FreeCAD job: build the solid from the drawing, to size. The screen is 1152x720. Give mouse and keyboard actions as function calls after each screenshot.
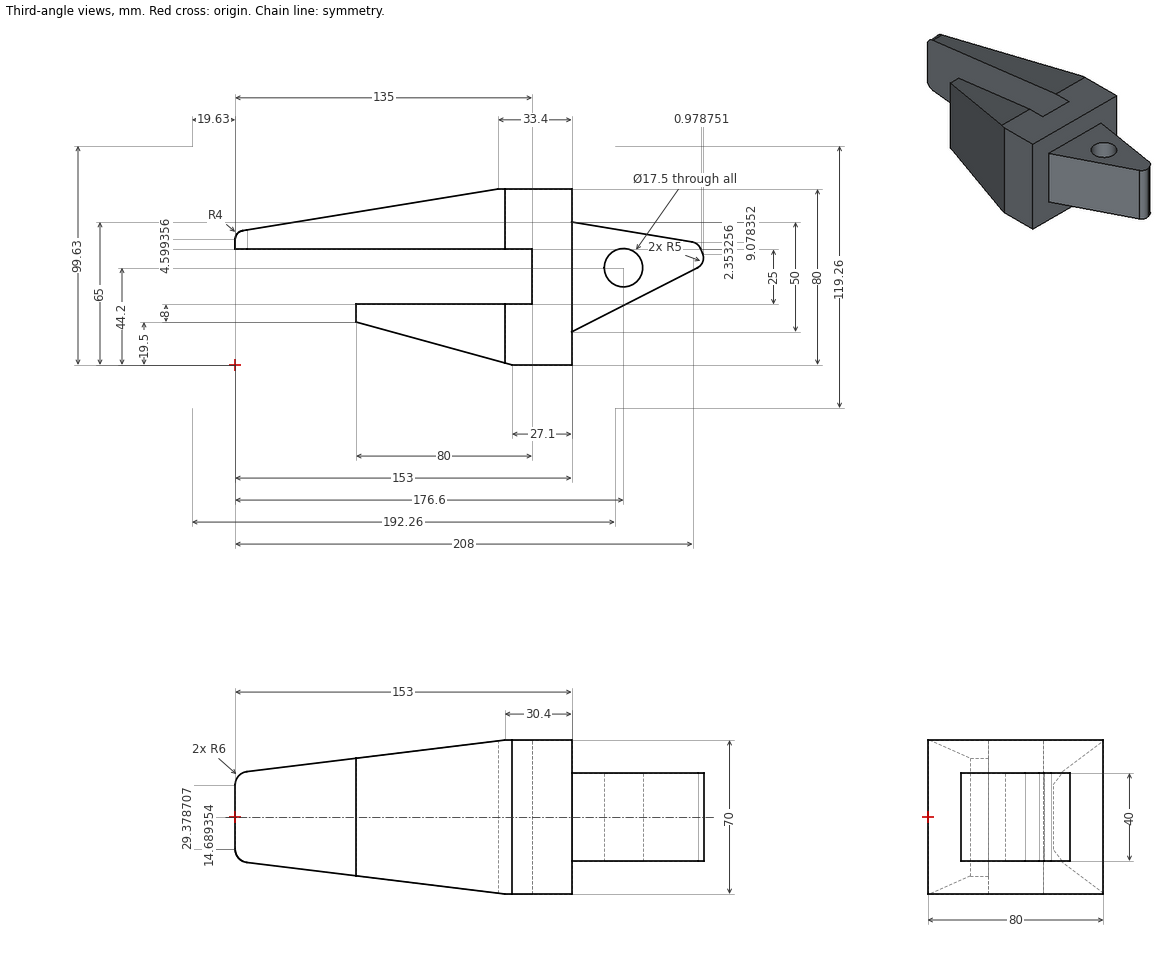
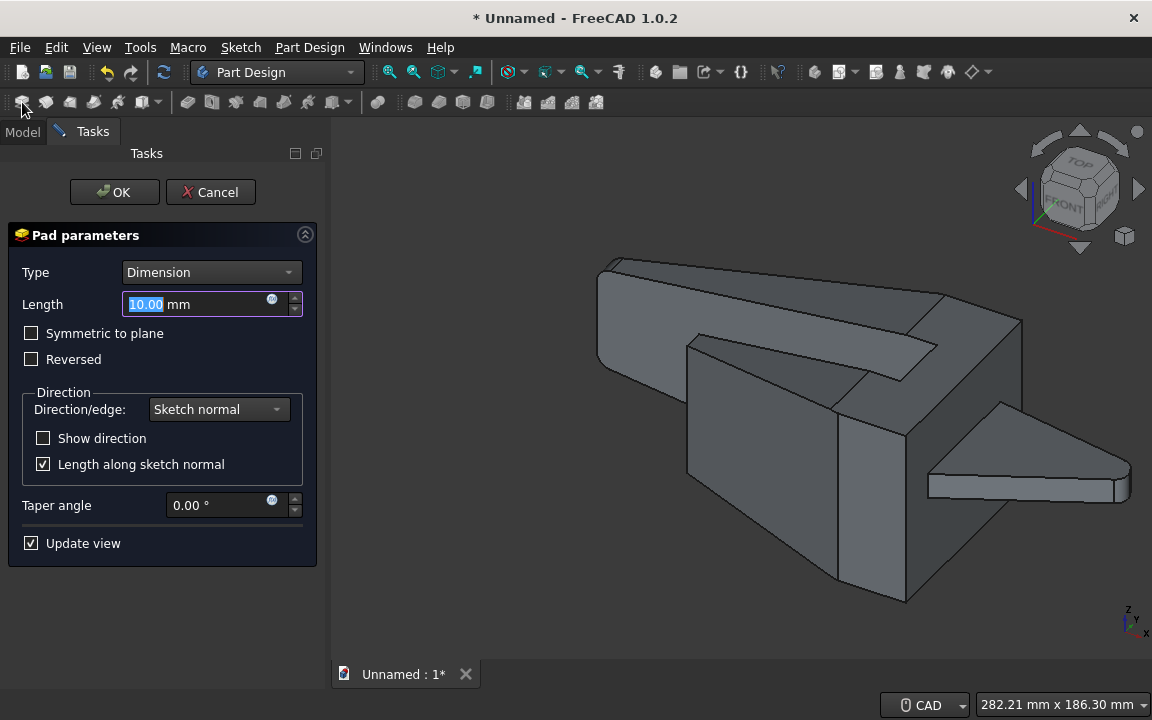
text(40)
key(Tab)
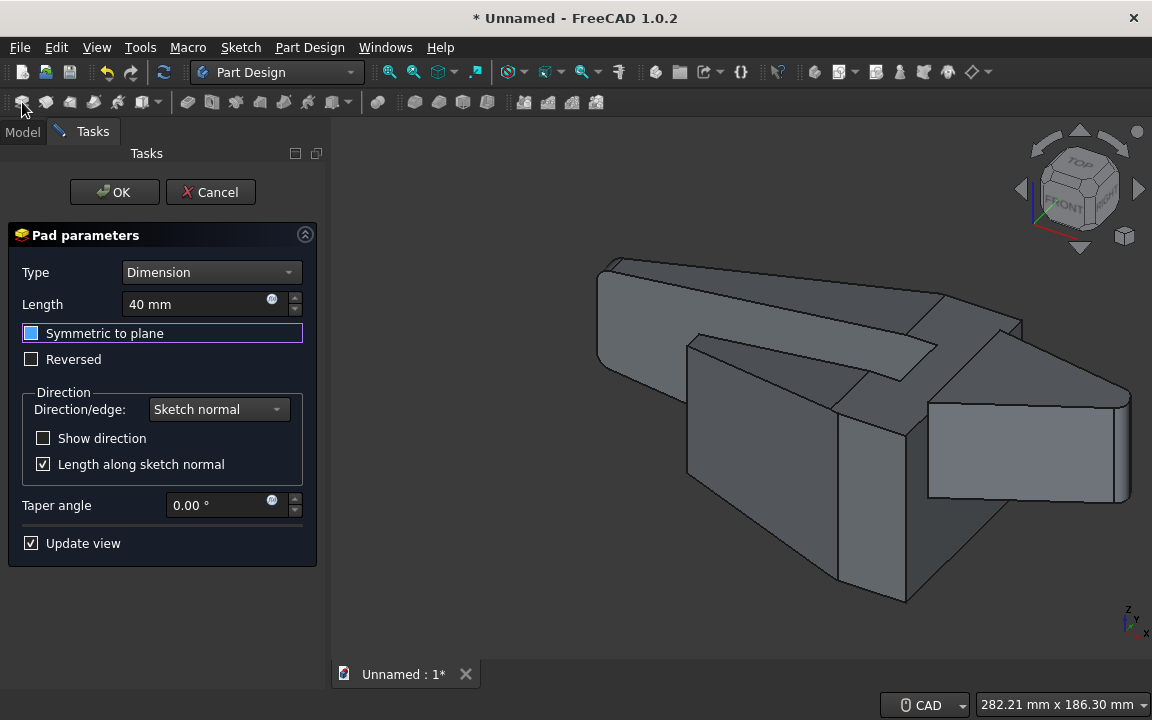
click(30, 333)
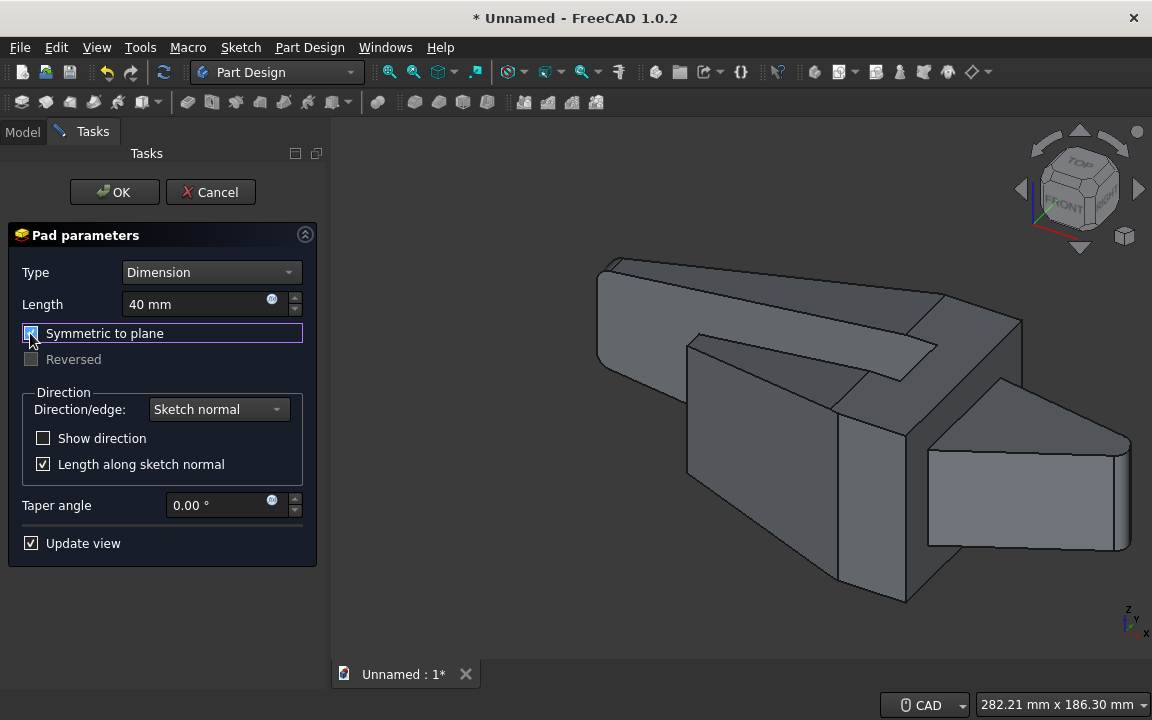
click(115, 192)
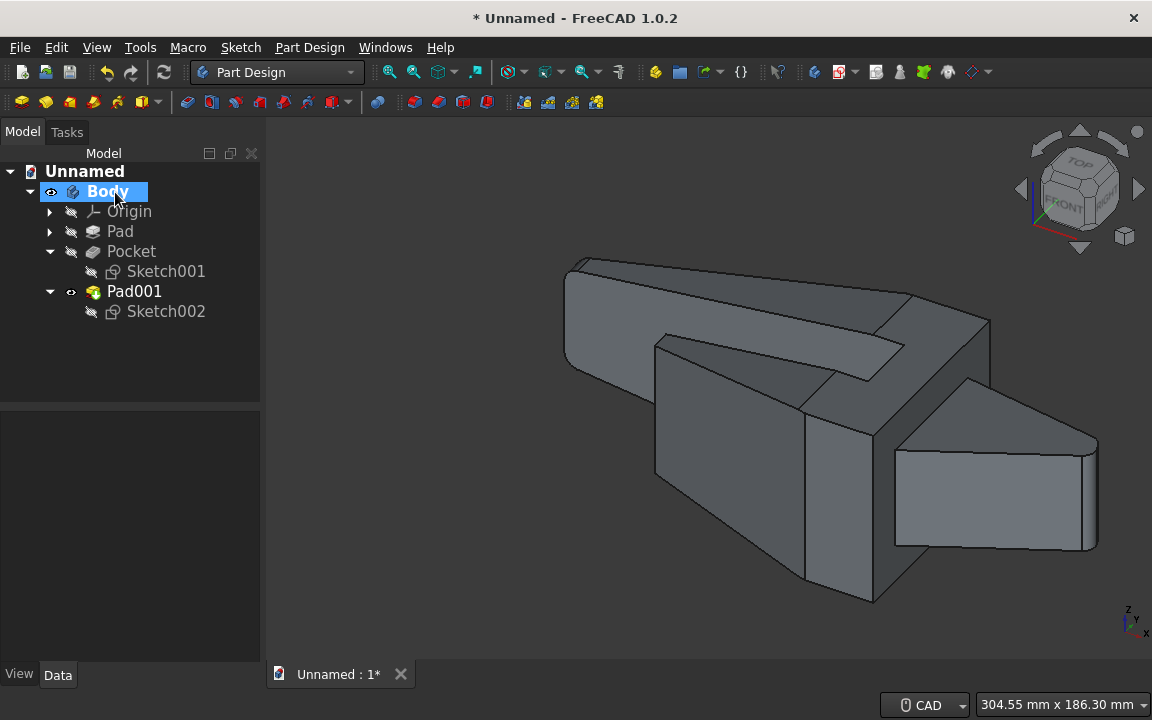
click(996, 421)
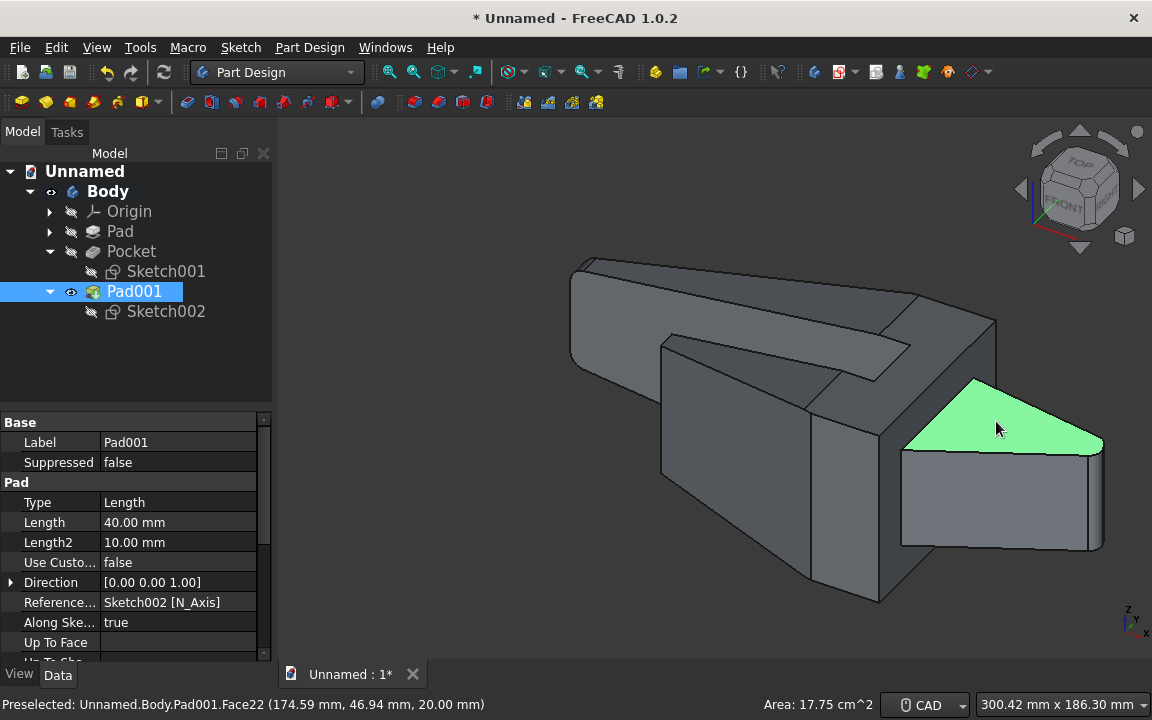
click(840, 72)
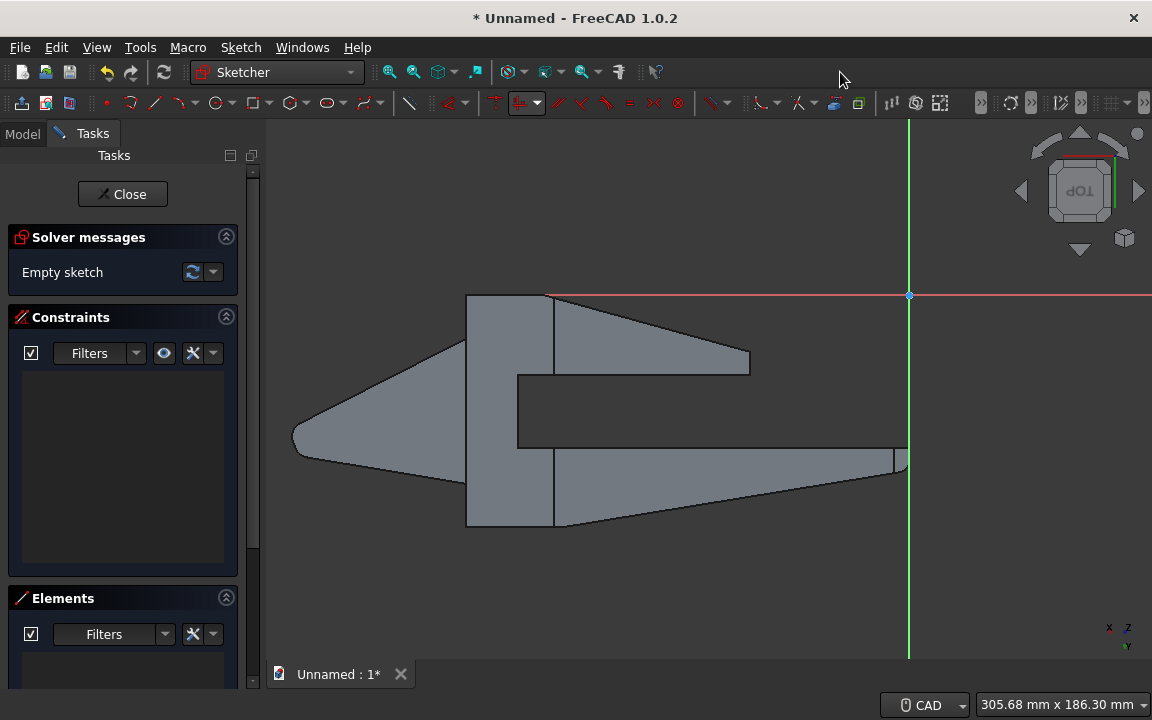
key(q)
key(s)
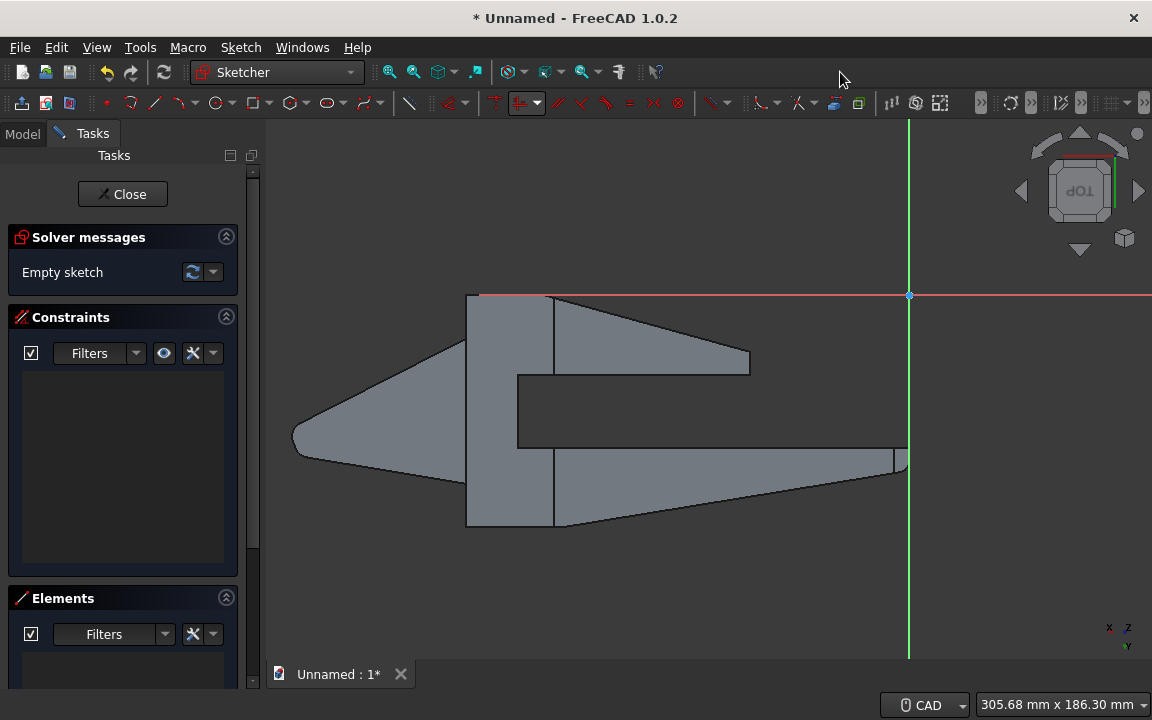
scroll(359, 429, up, 10)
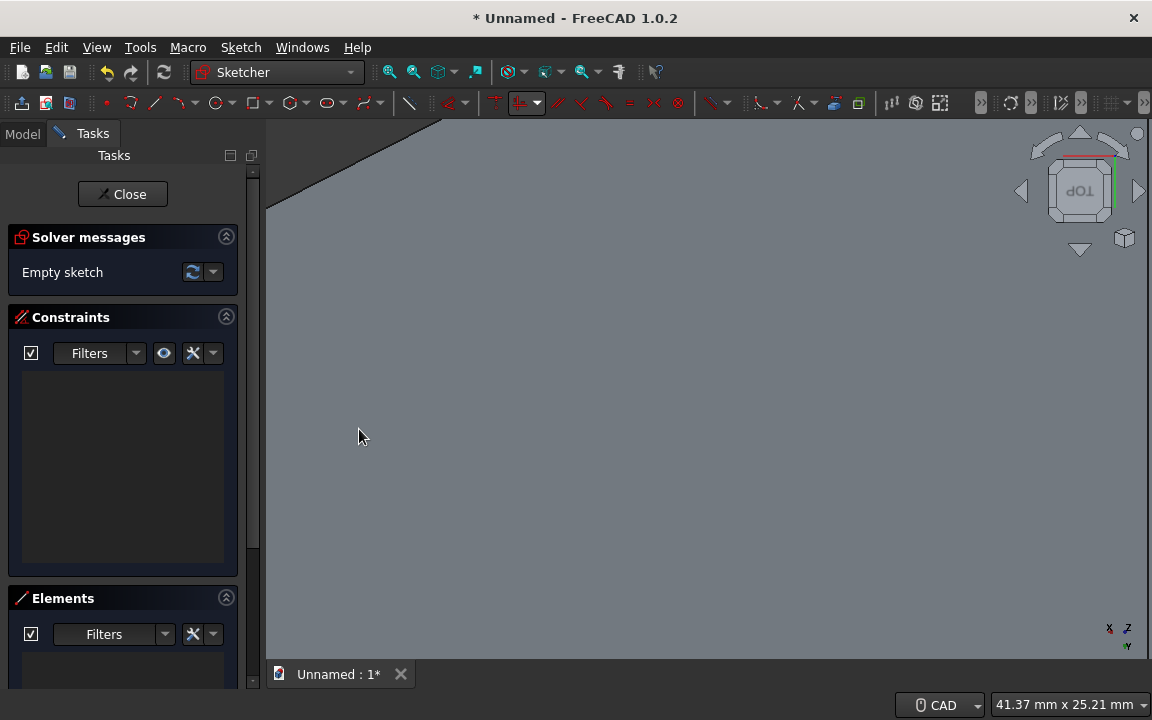
click(216, 104)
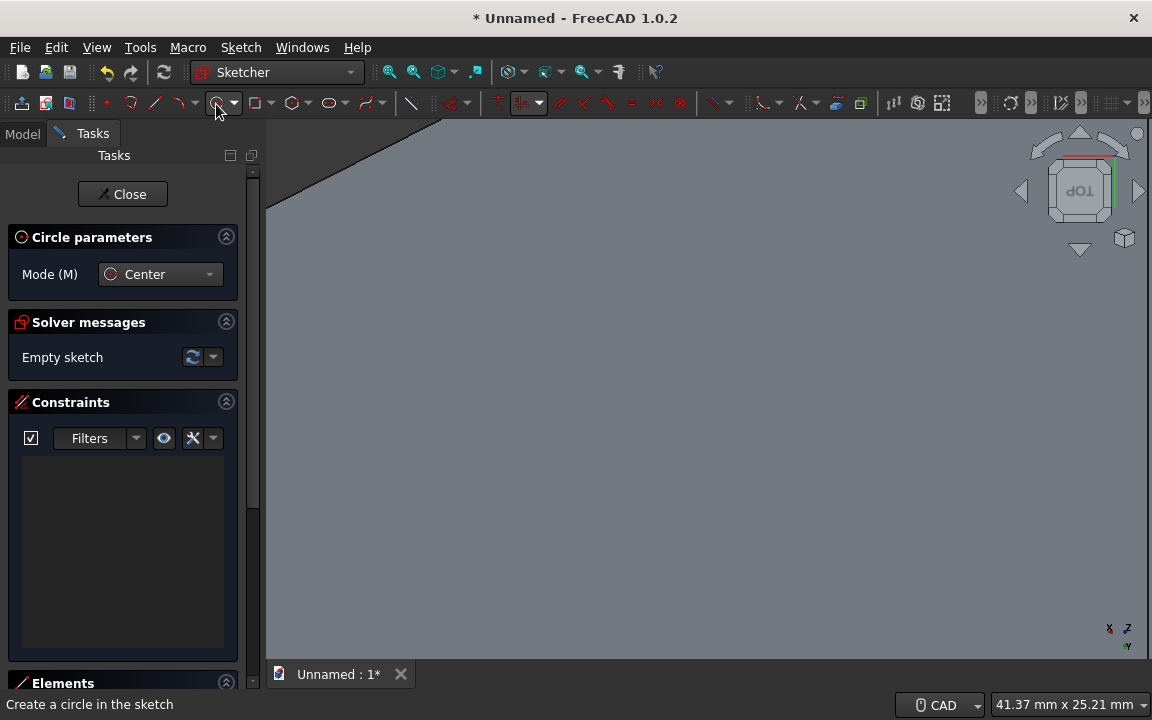
click(643, 385)
move(775, 252)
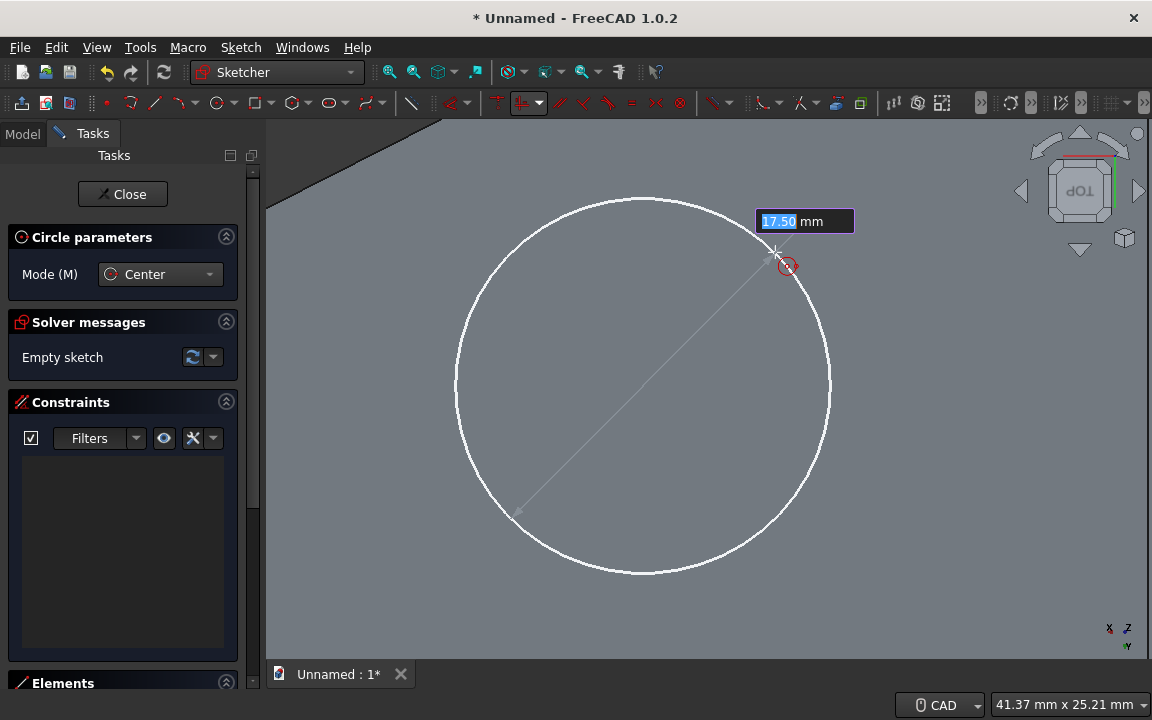
text(17.5)
key(Return)
key(Escape)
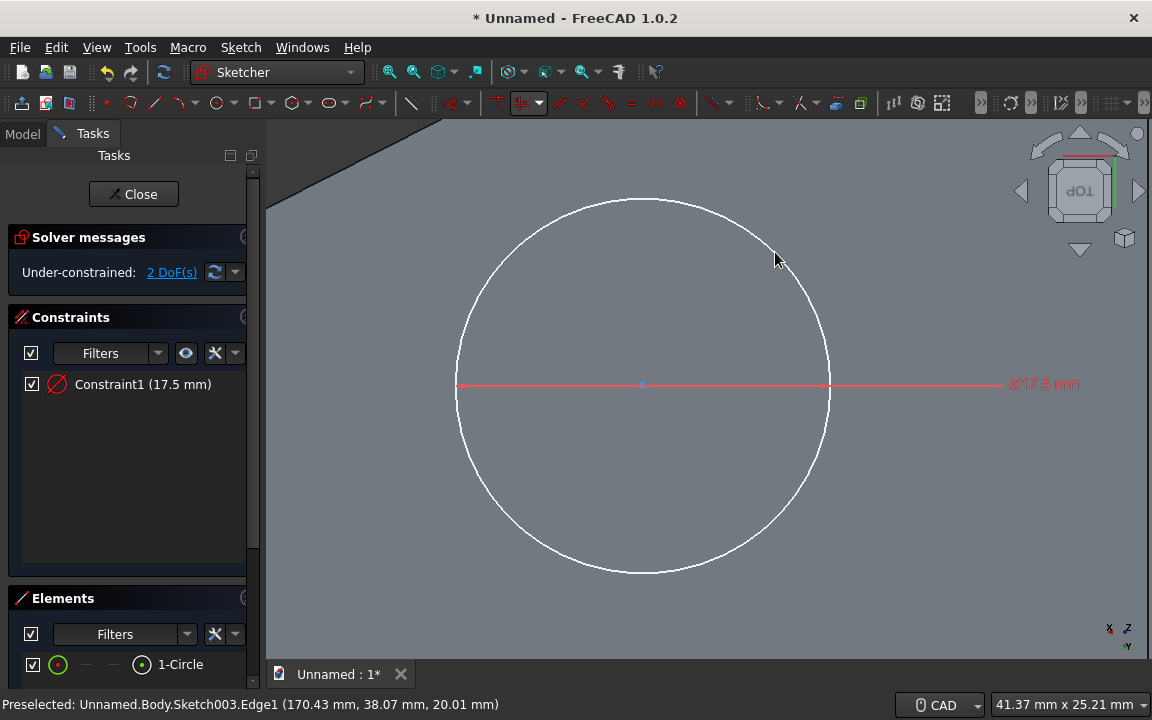
key(d)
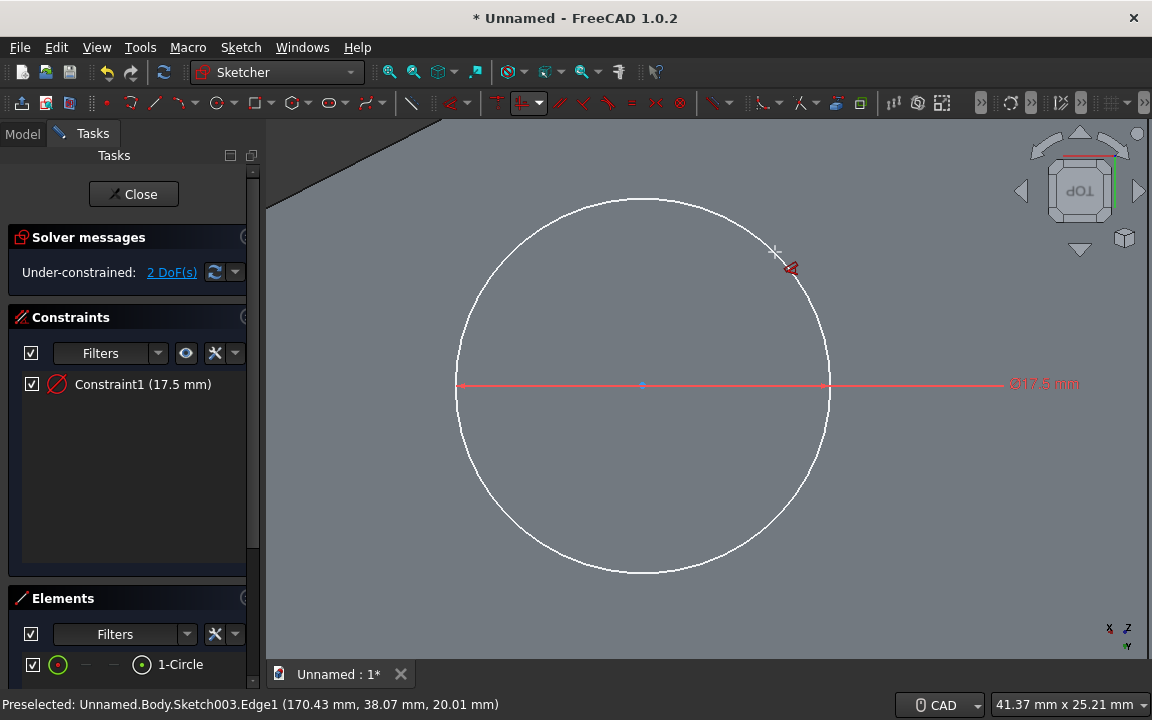
click(643, 386)
click(609, 266)